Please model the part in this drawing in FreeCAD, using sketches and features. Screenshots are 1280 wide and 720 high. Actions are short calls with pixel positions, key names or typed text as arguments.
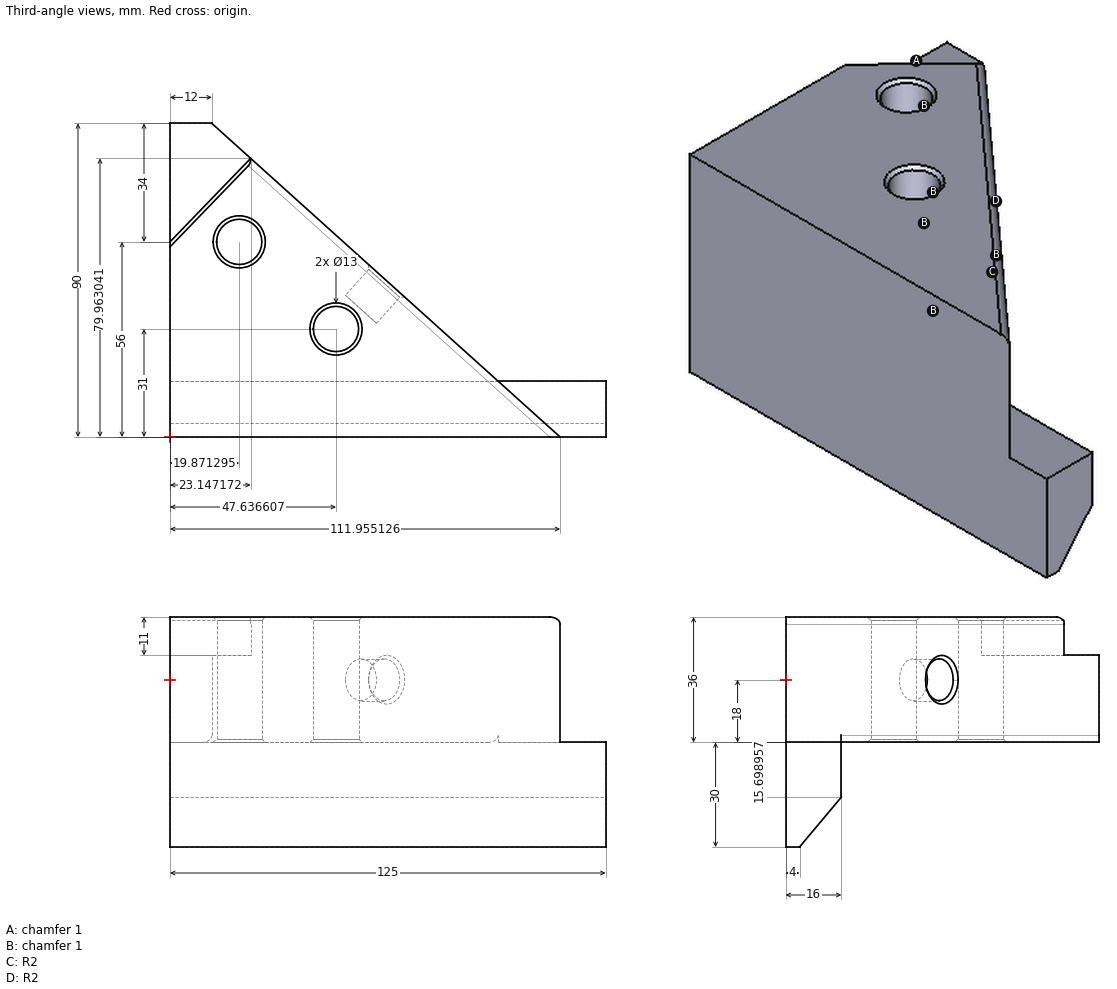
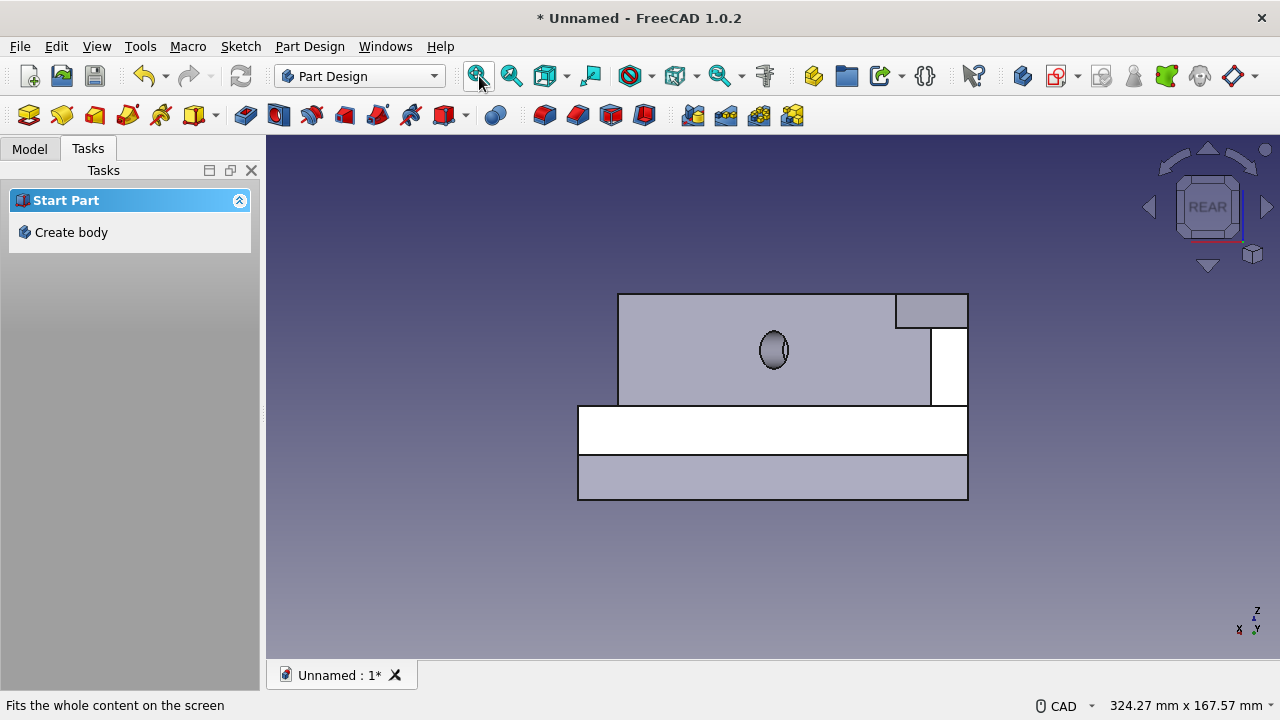
key(5)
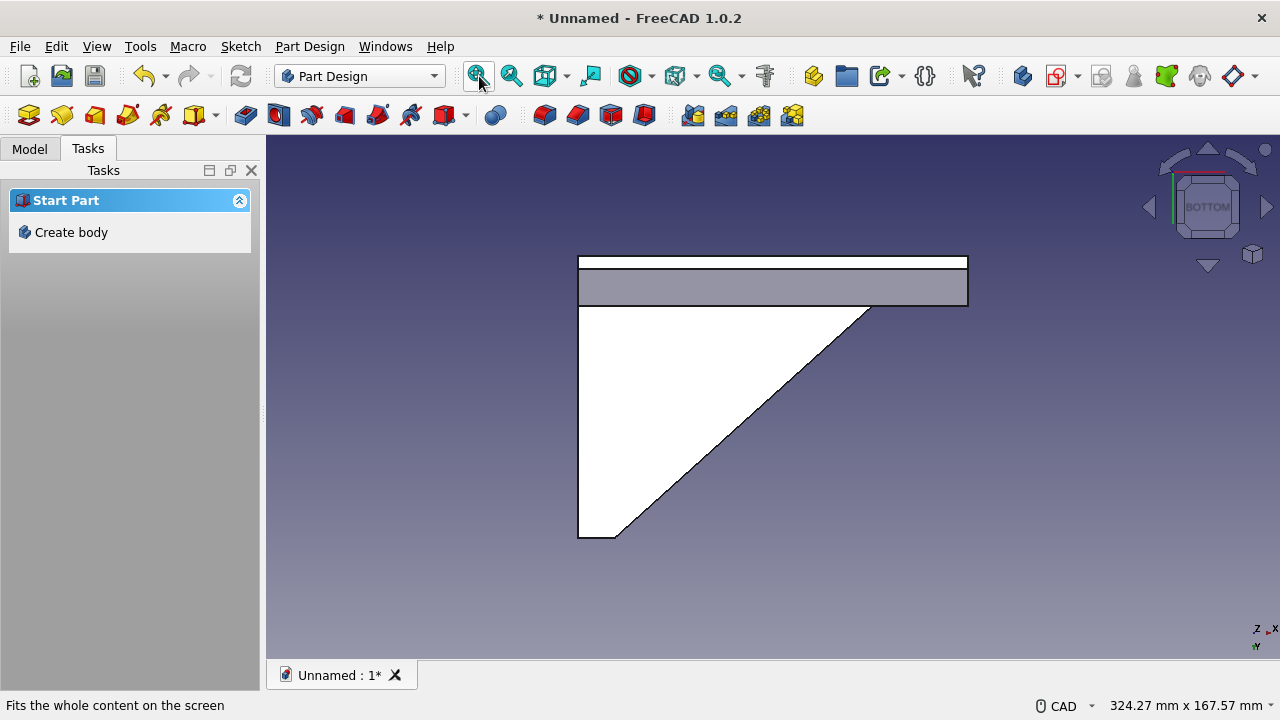
click(683, 388)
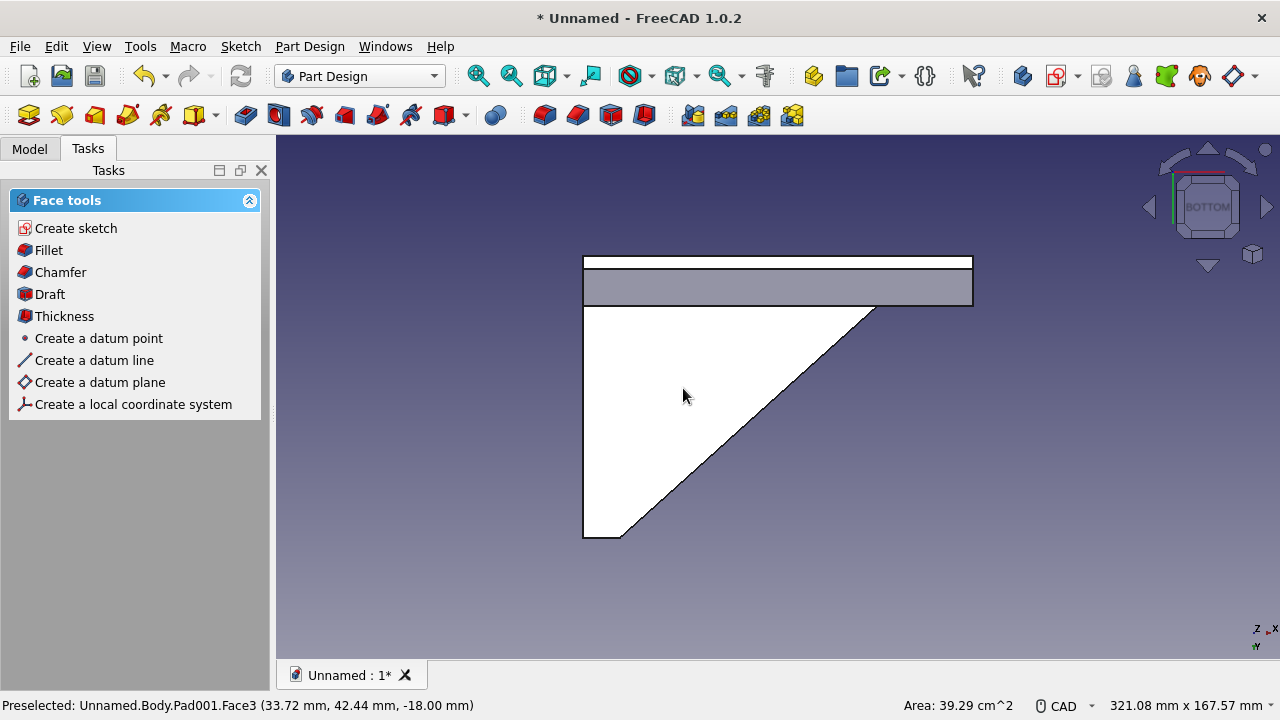
click(1056, 76)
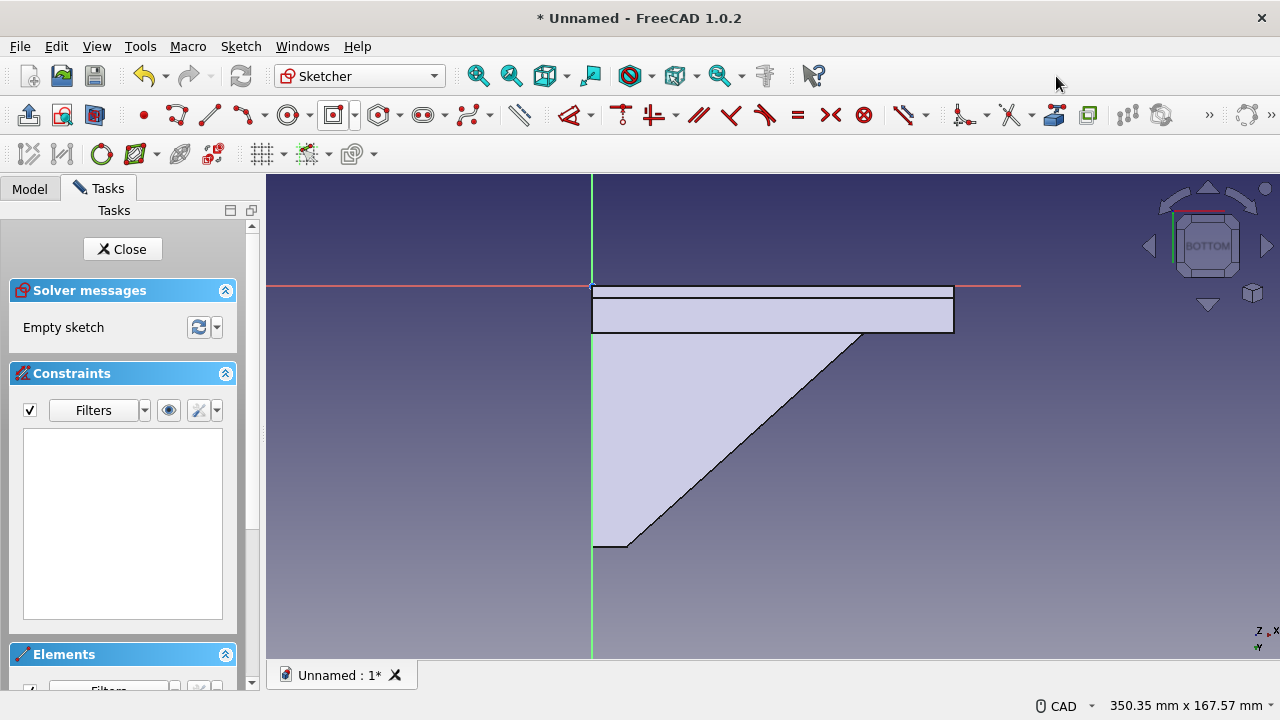
click(95, 116)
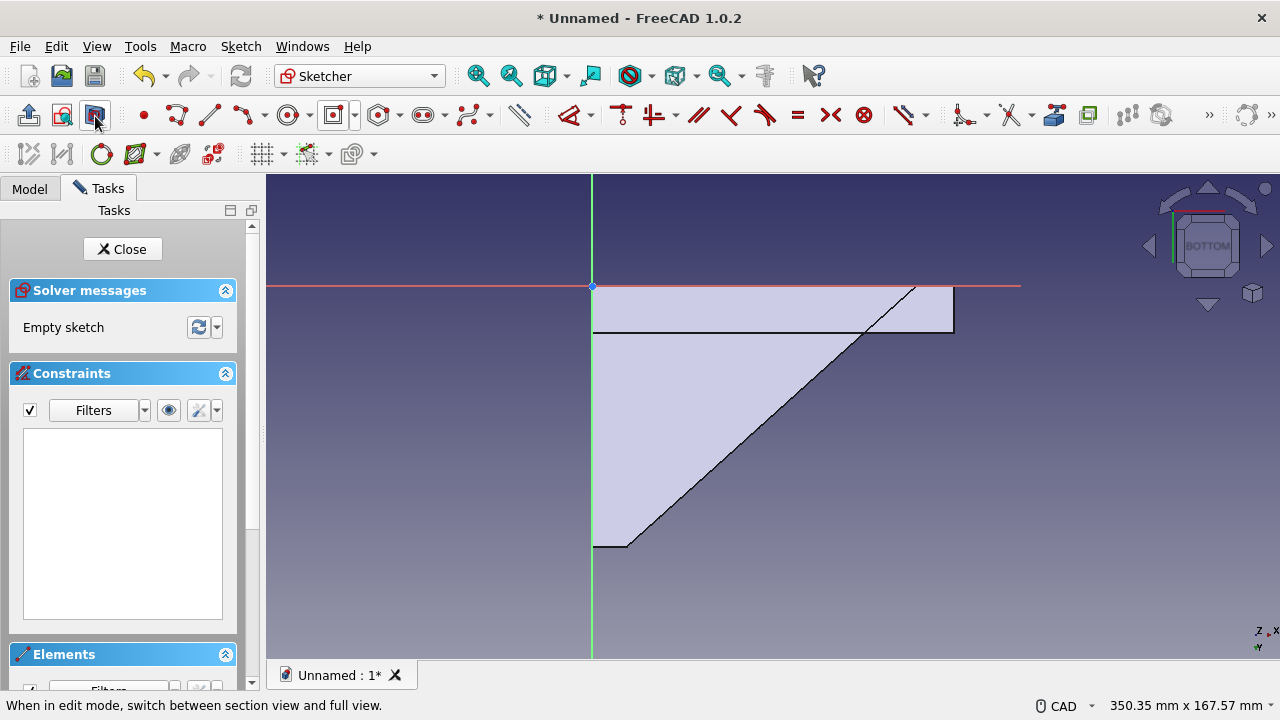
scroll(629, 328, up, 3)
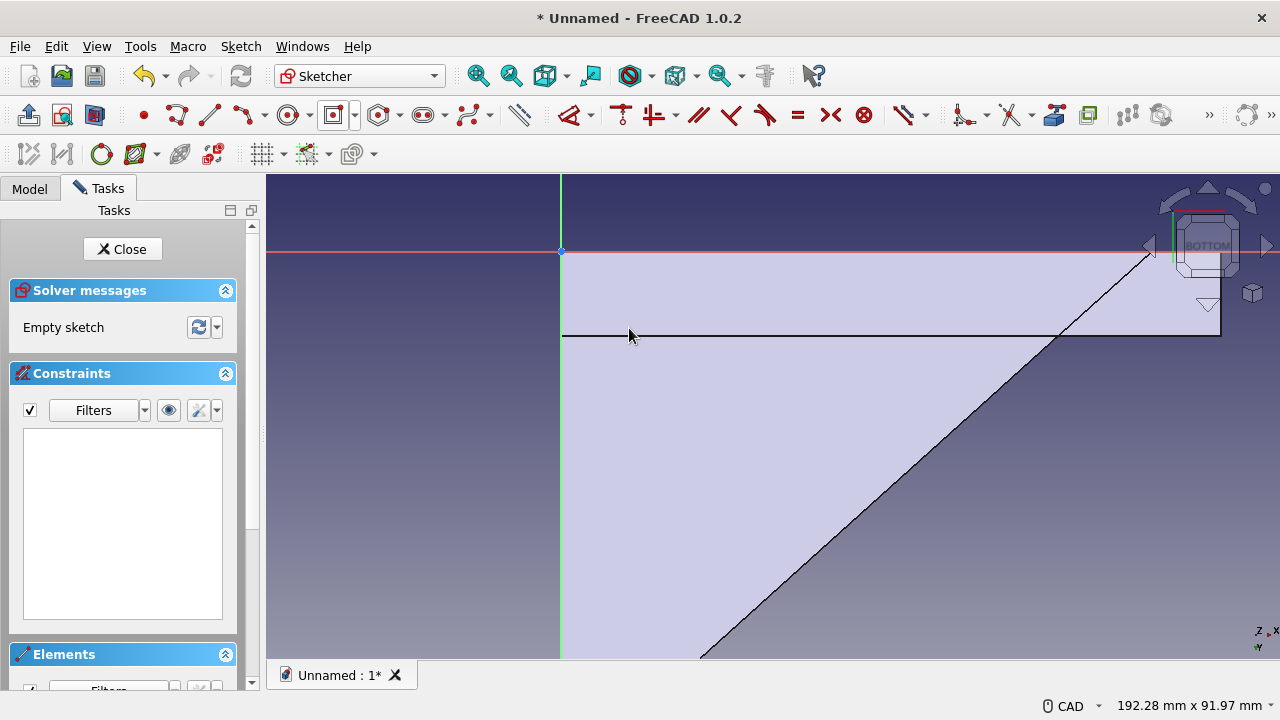
click(288, 116)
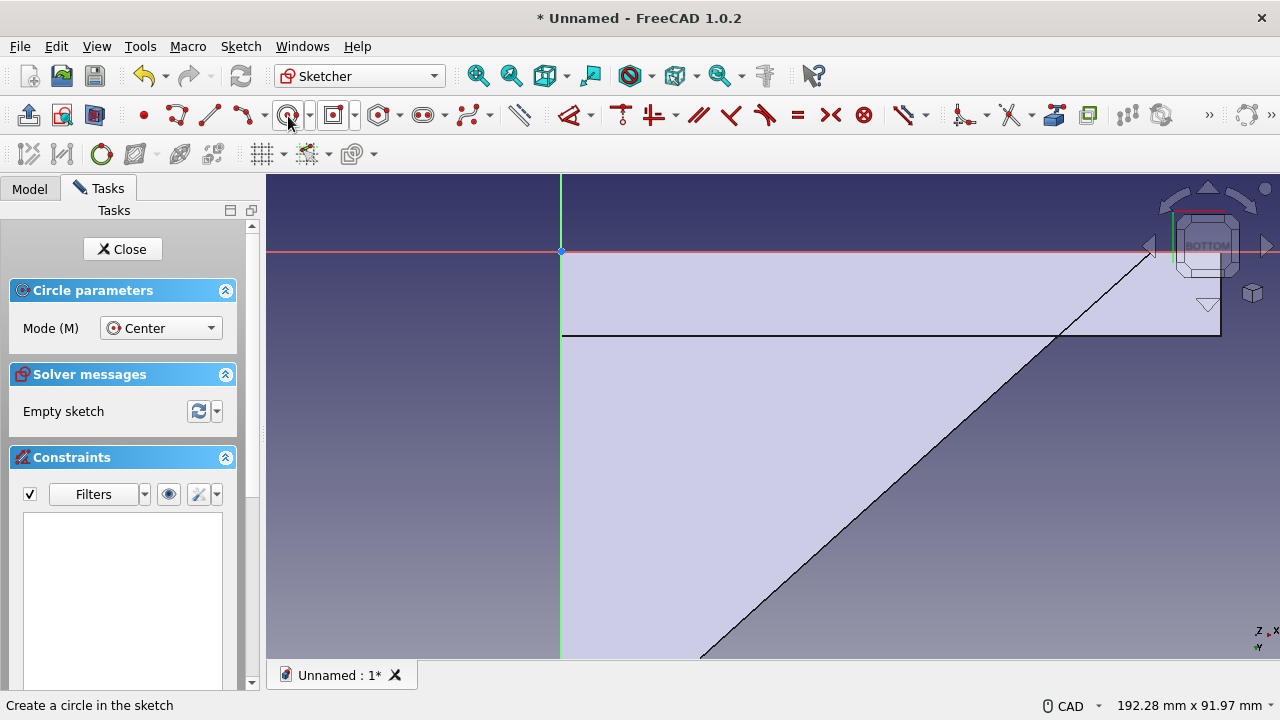
click(813, 415)
click(837, 391)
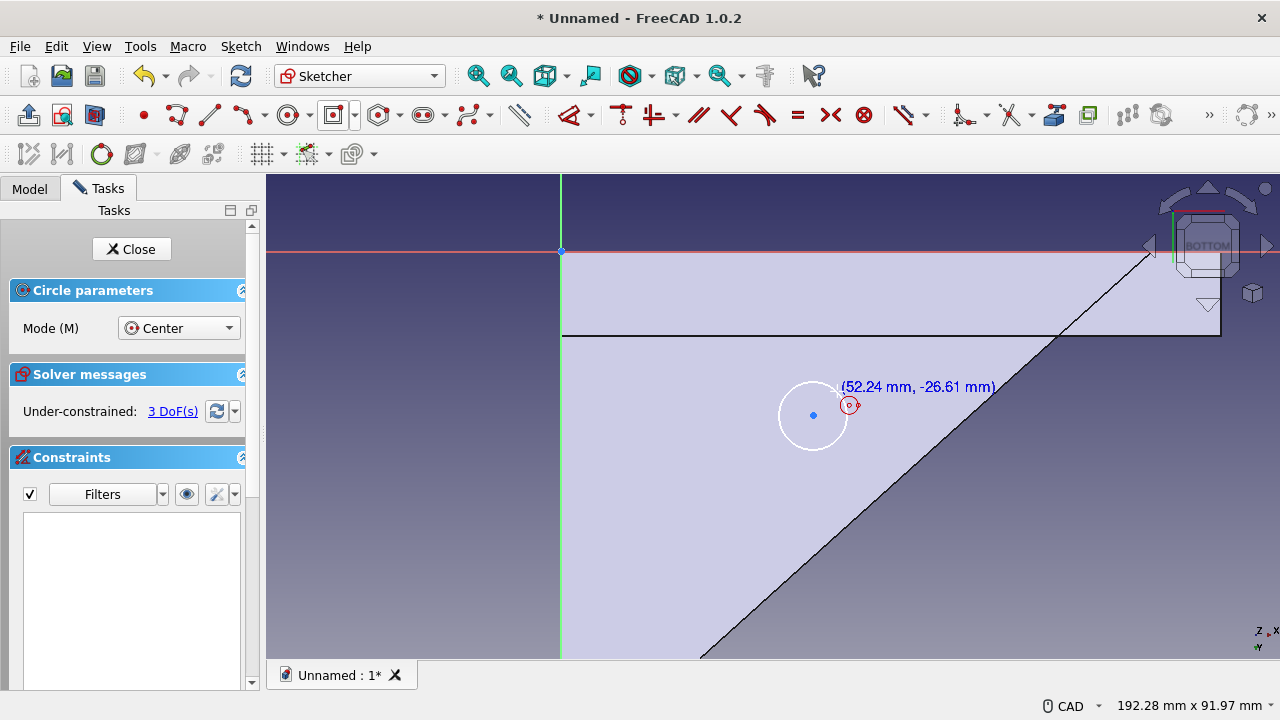
click(666, 547)
click(691, 523)
key(Escape)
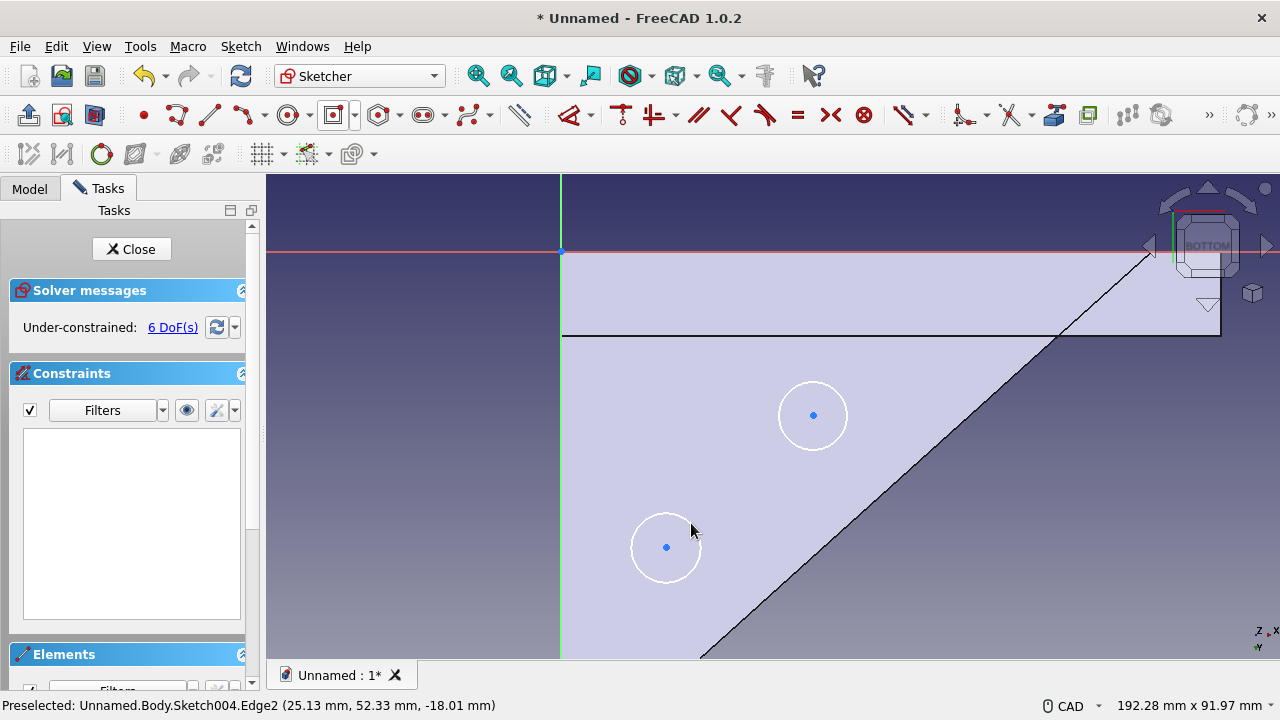
click(837, 392)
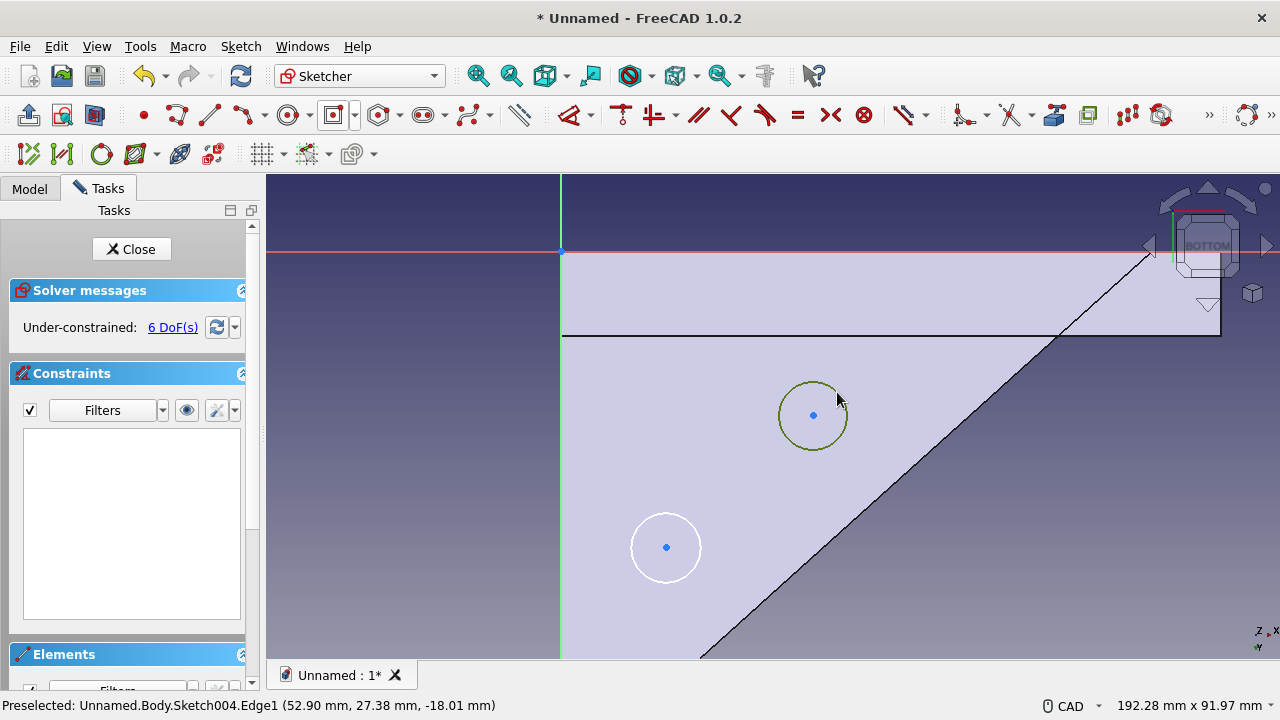
click(690, 523)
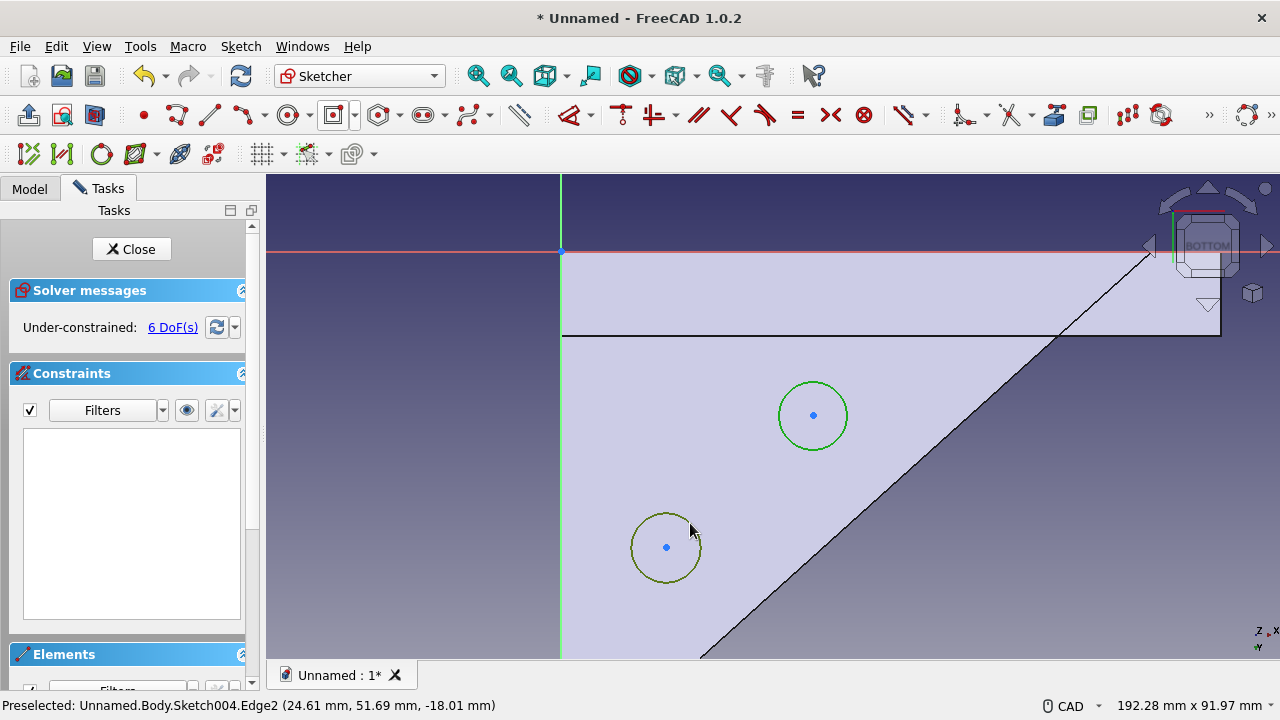
key(e)